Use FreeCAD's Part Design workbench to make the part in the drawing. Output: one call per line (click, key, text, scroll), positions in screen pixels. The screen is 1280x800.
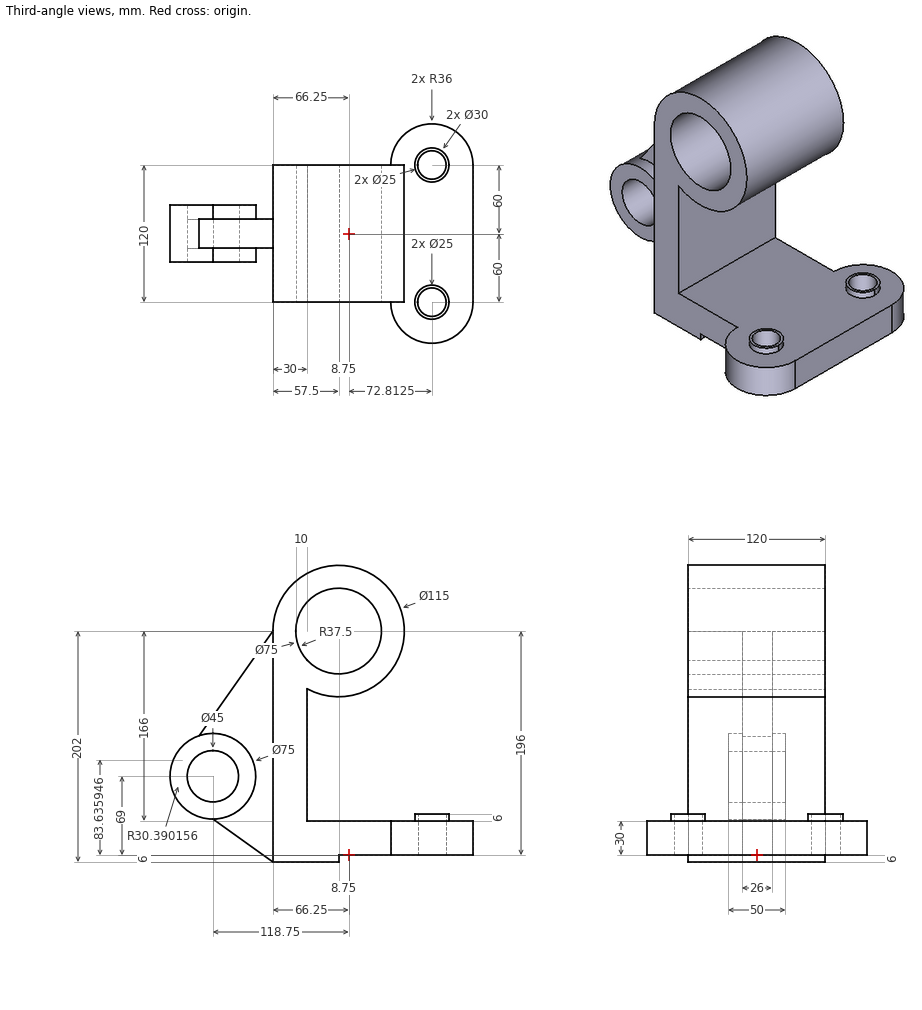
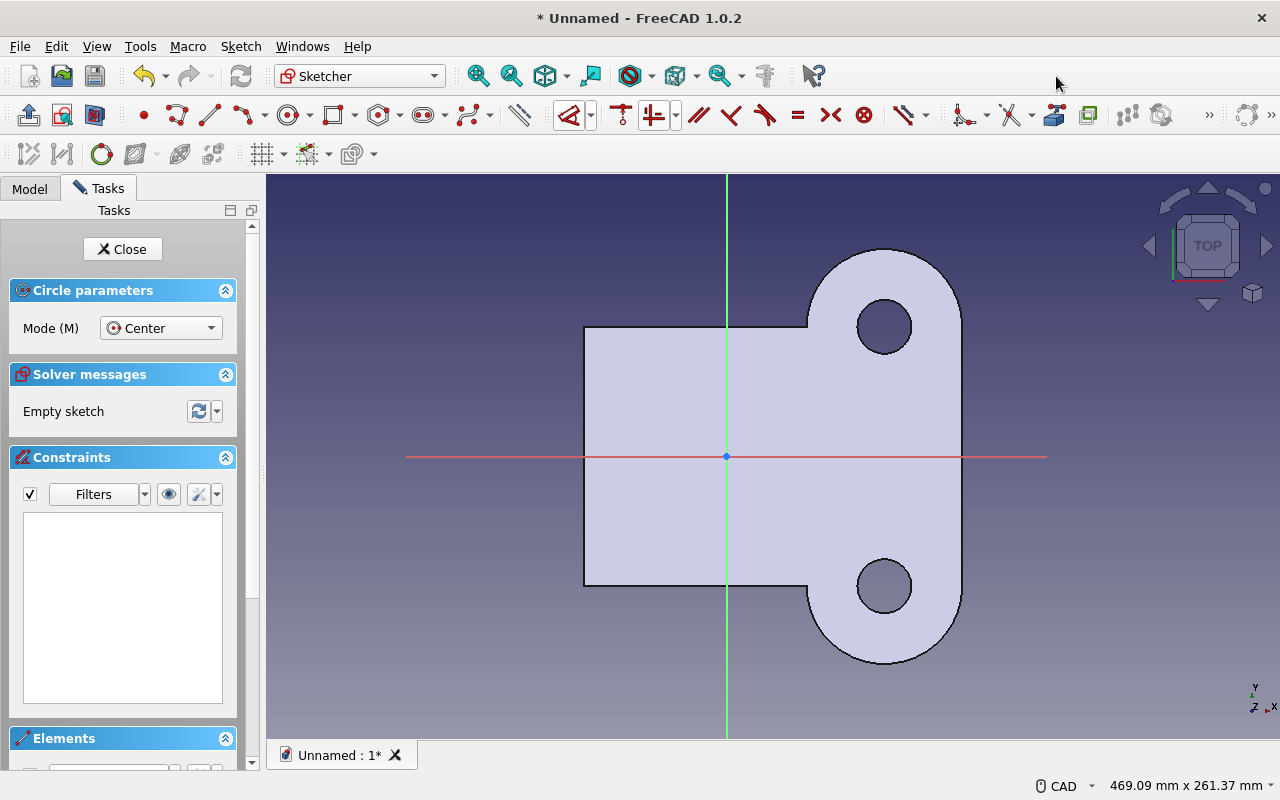
click(884, 327)
click(907, 304)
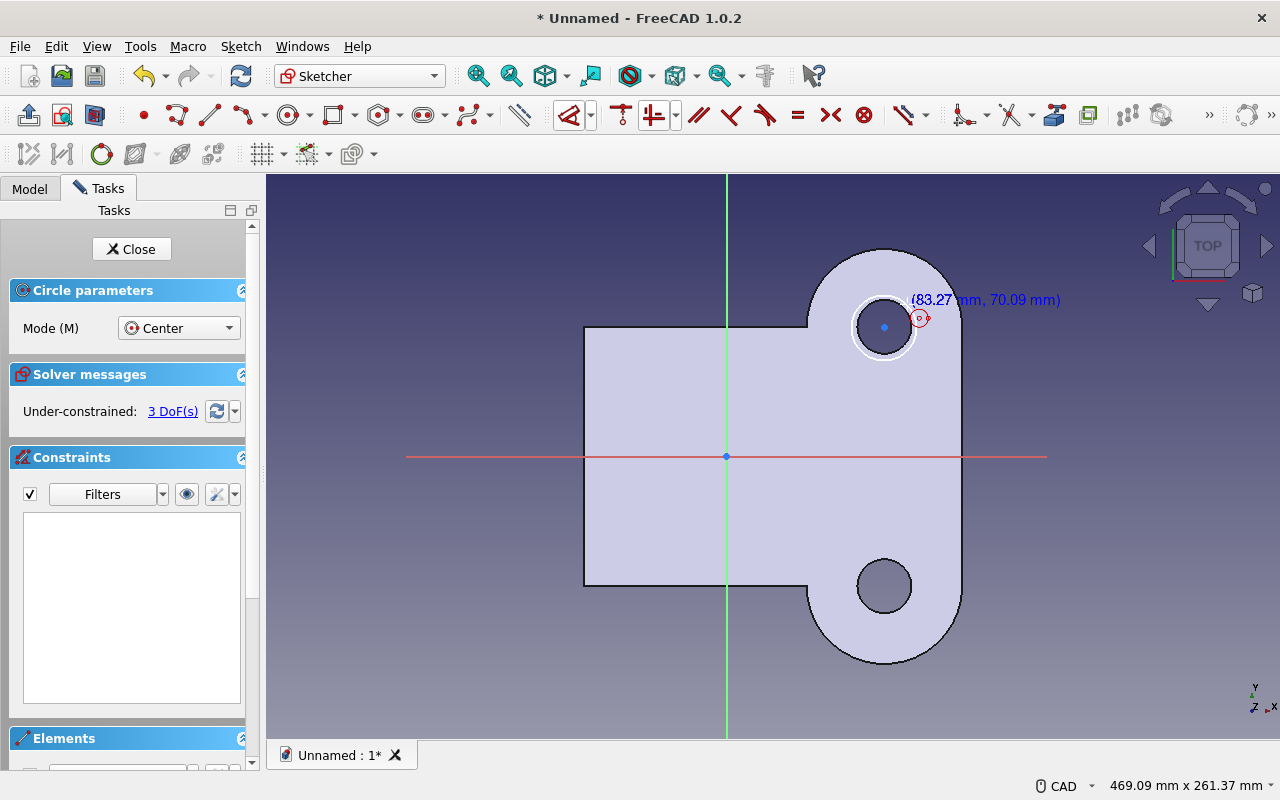
click(884, 586)
click(907, 563)
key(Escape)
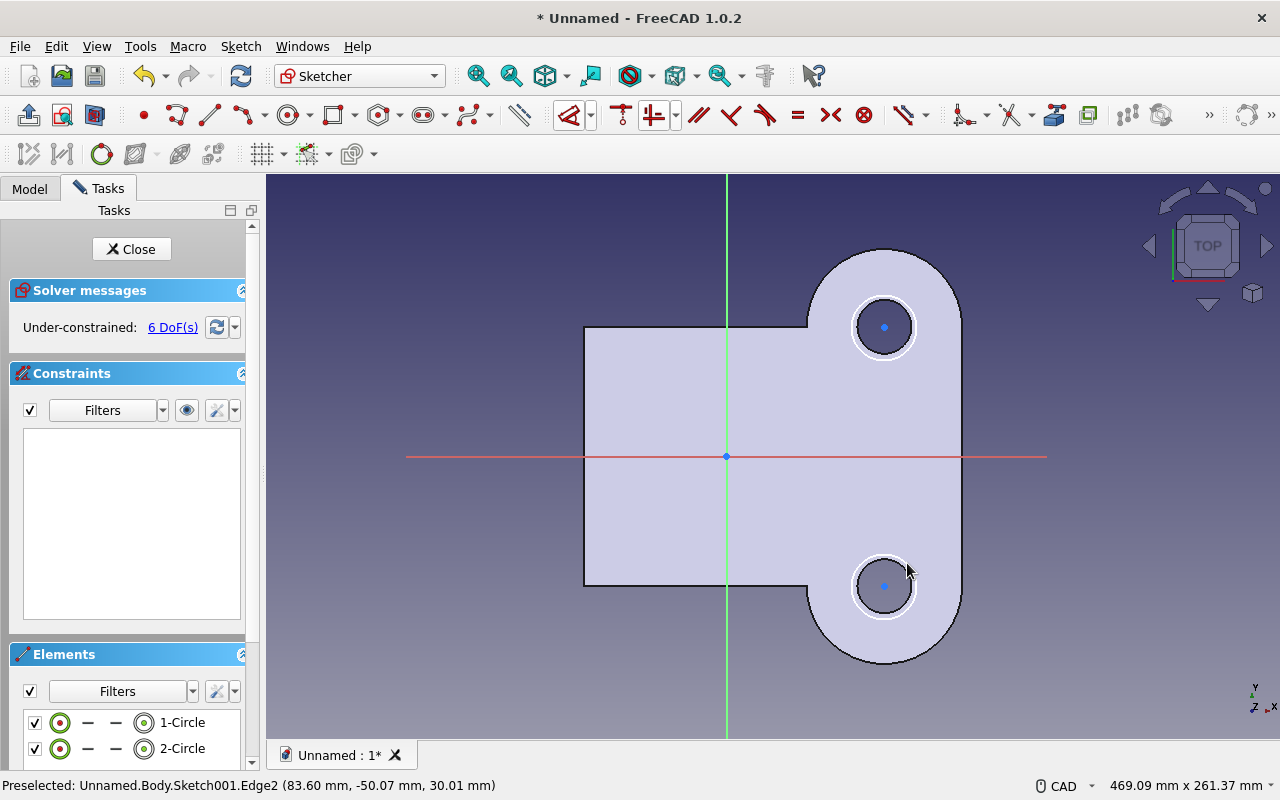
click(907, 305)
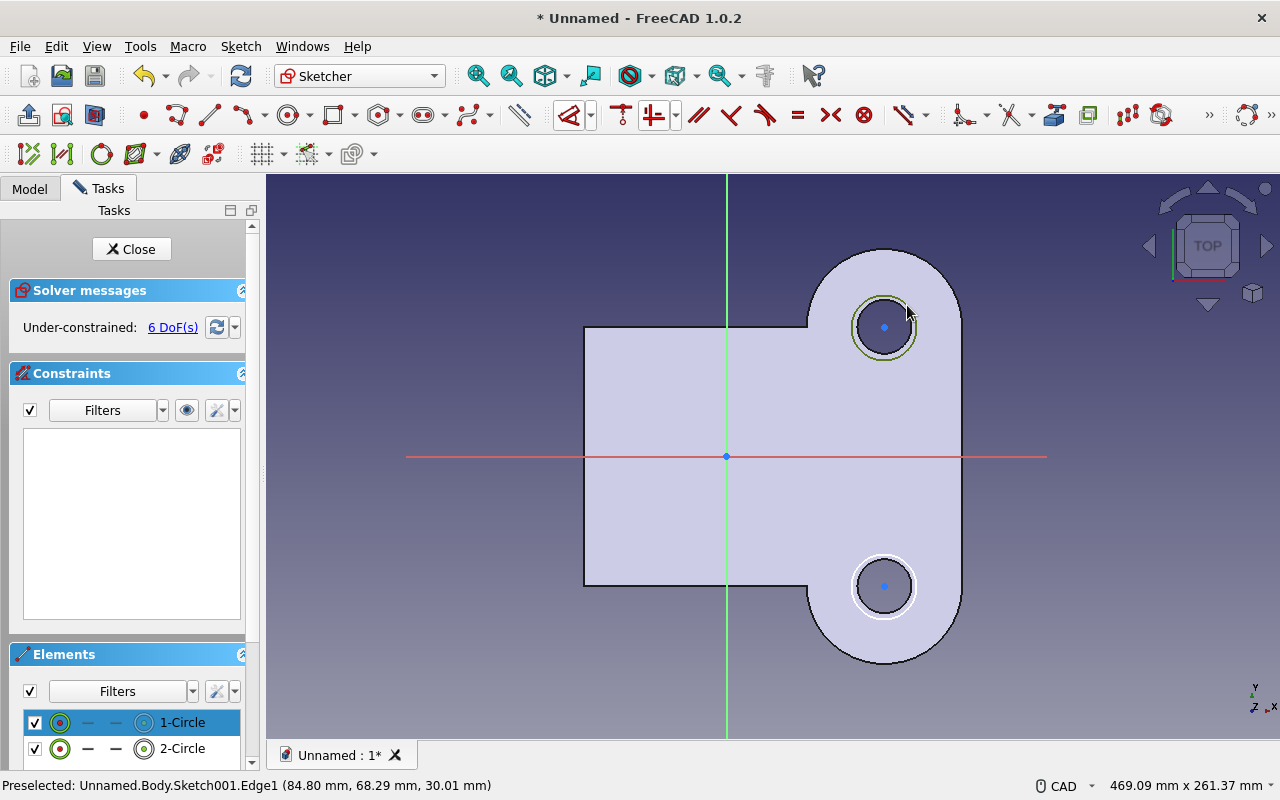
click(907, 564)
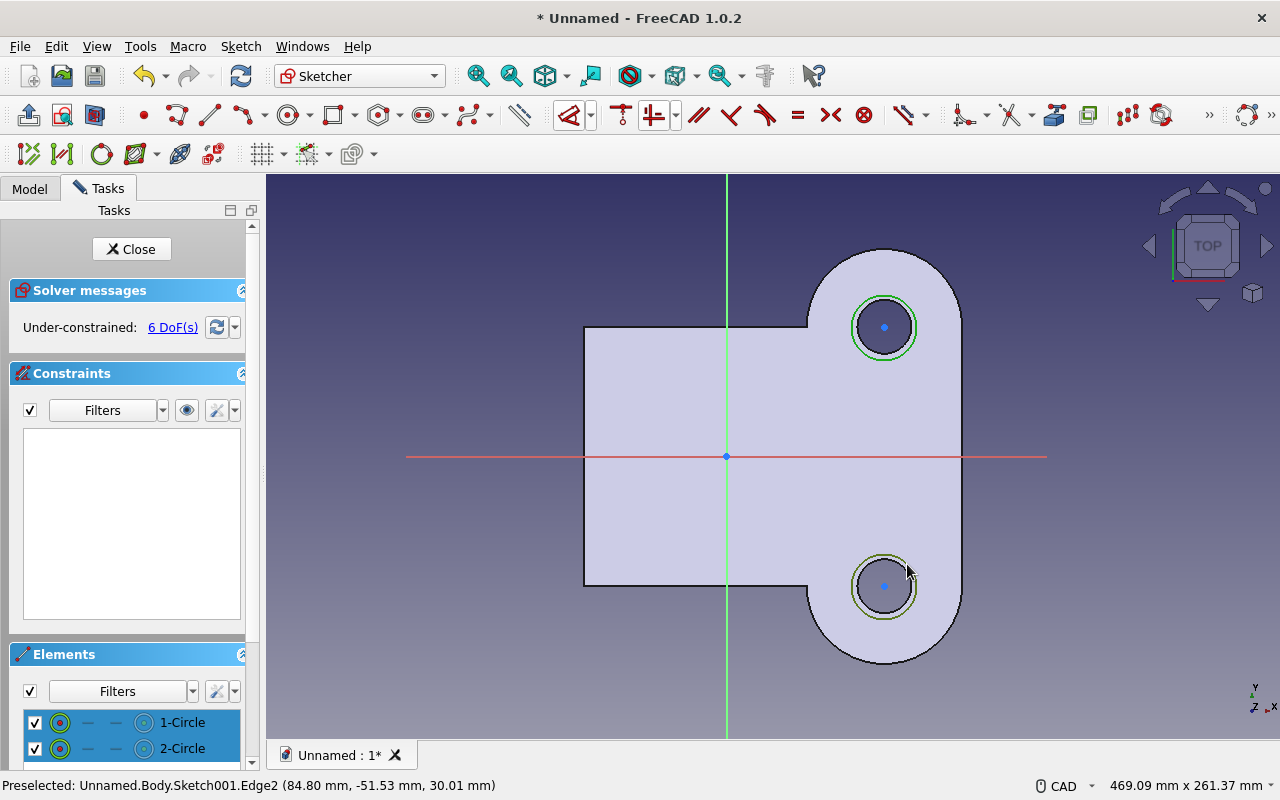
click(798, 116)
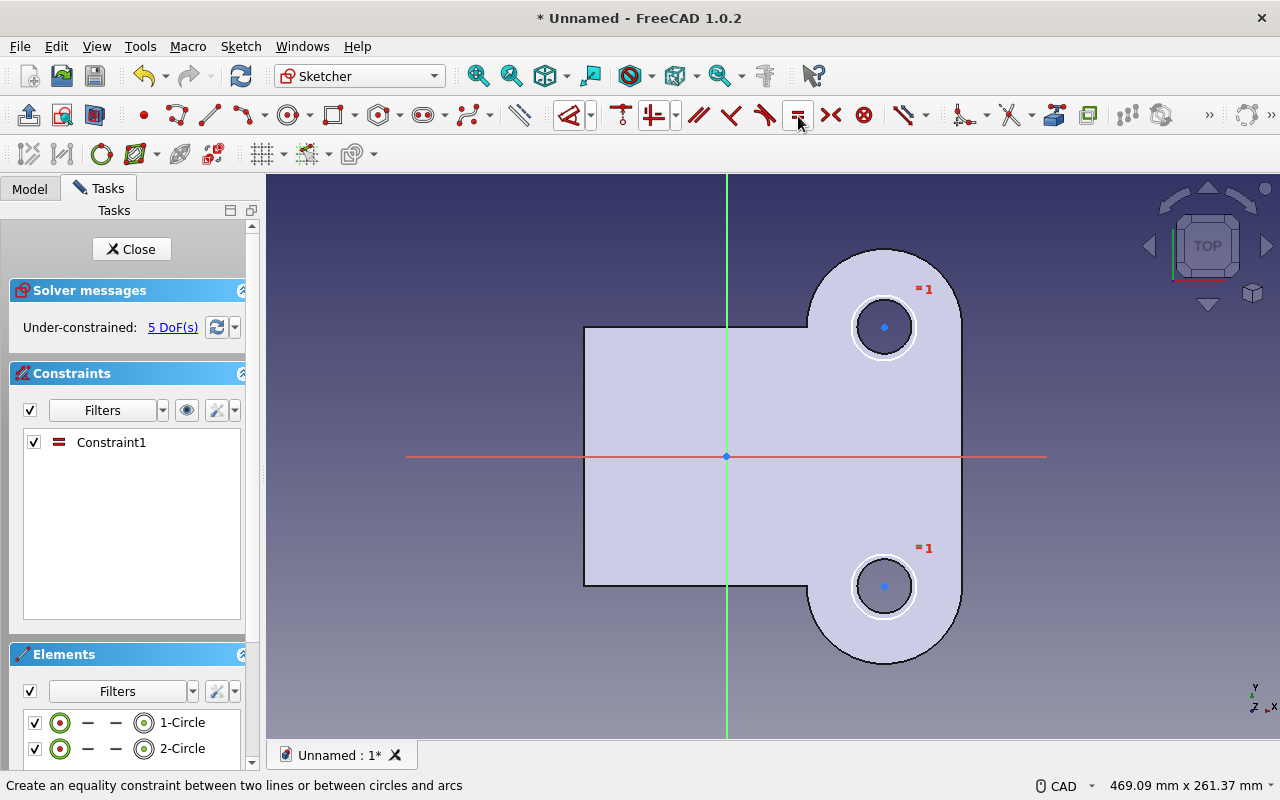
click(884, 328)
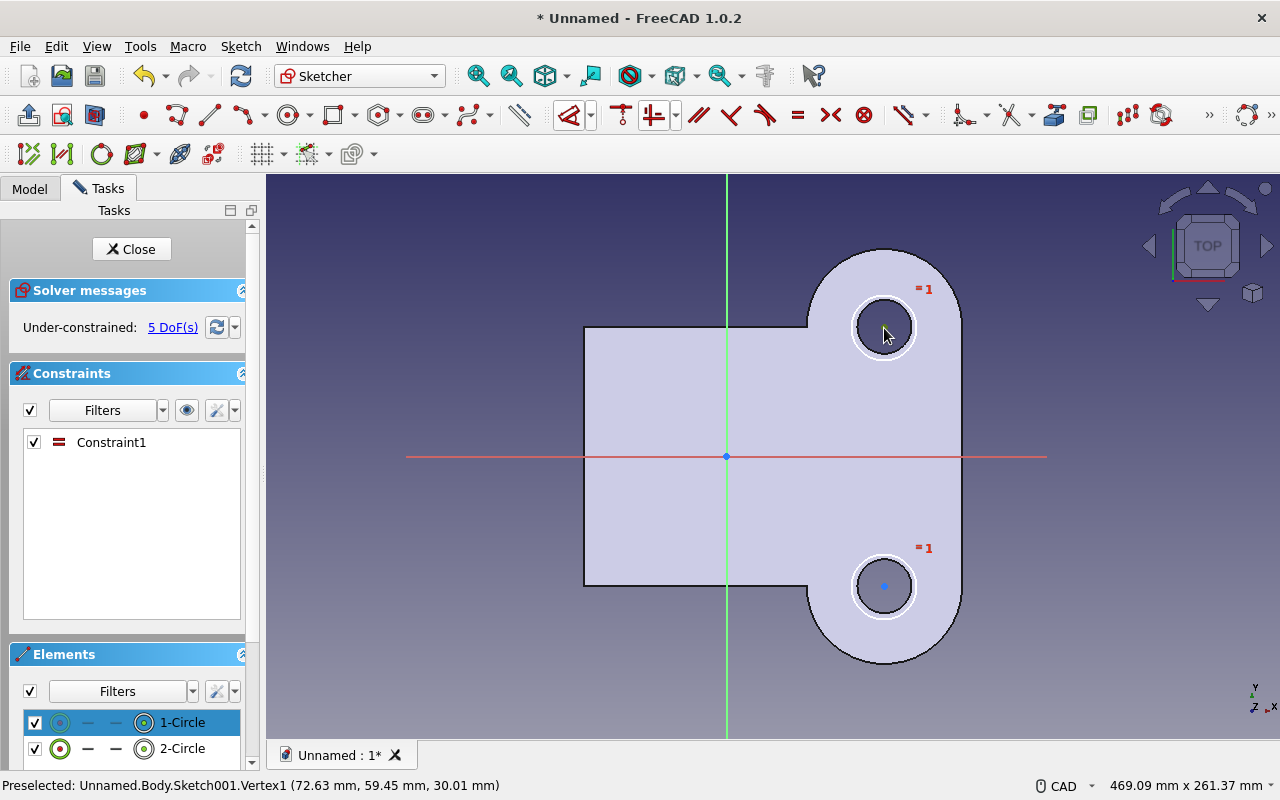
click(884, 587)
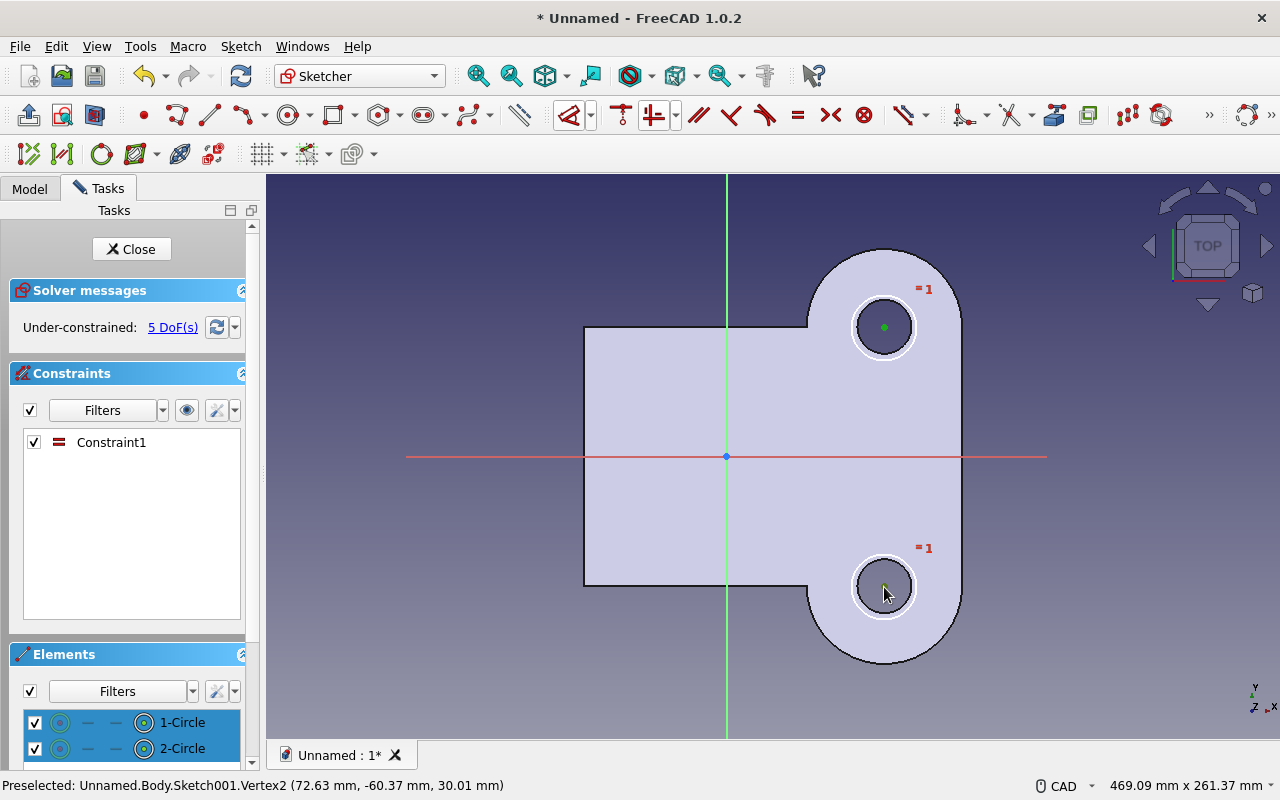
click(676, 116)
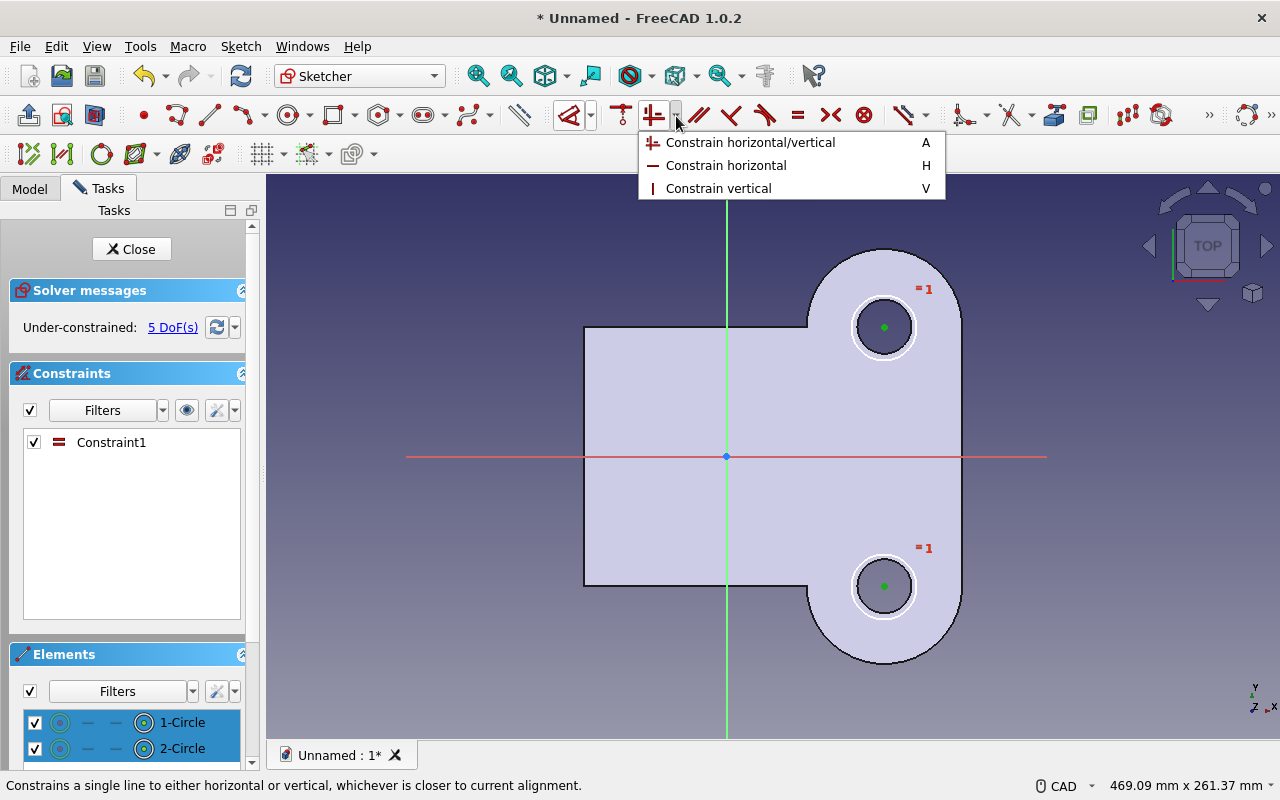
click(792, 188)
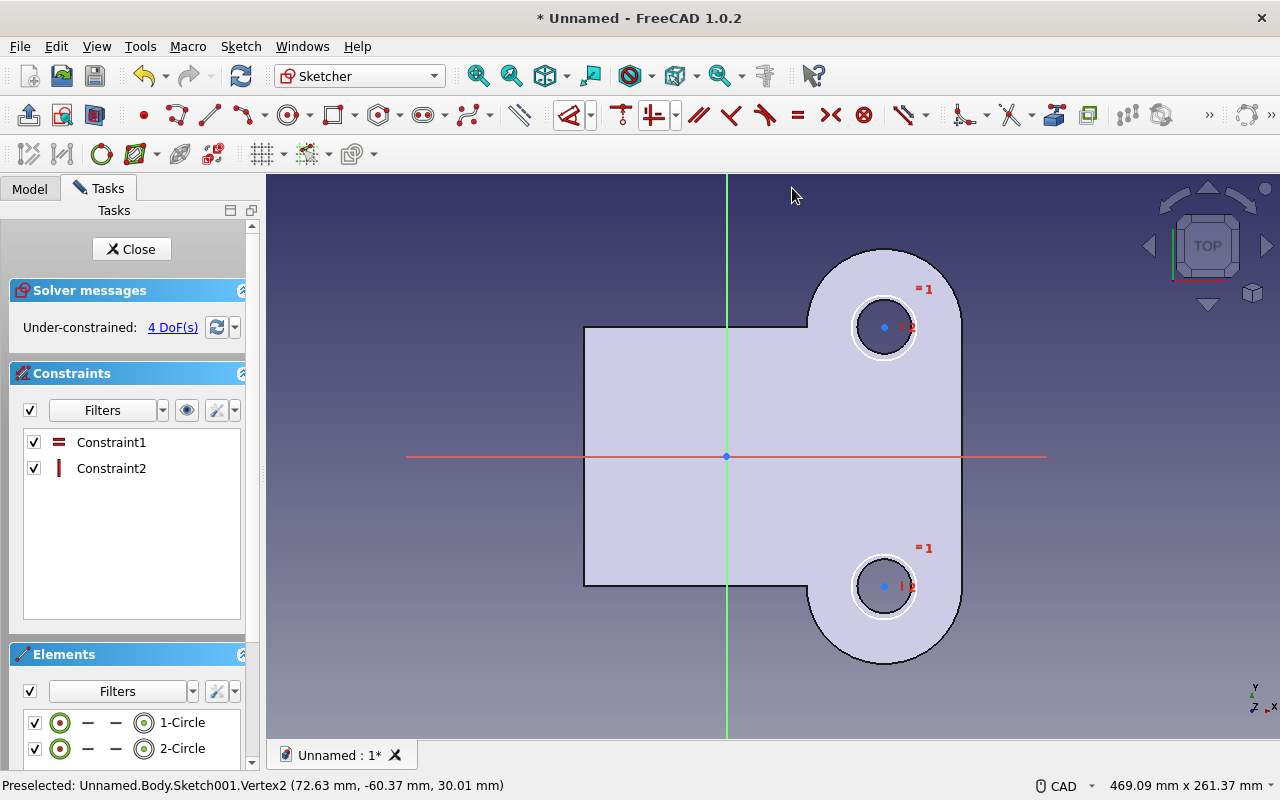
click(907, 305)